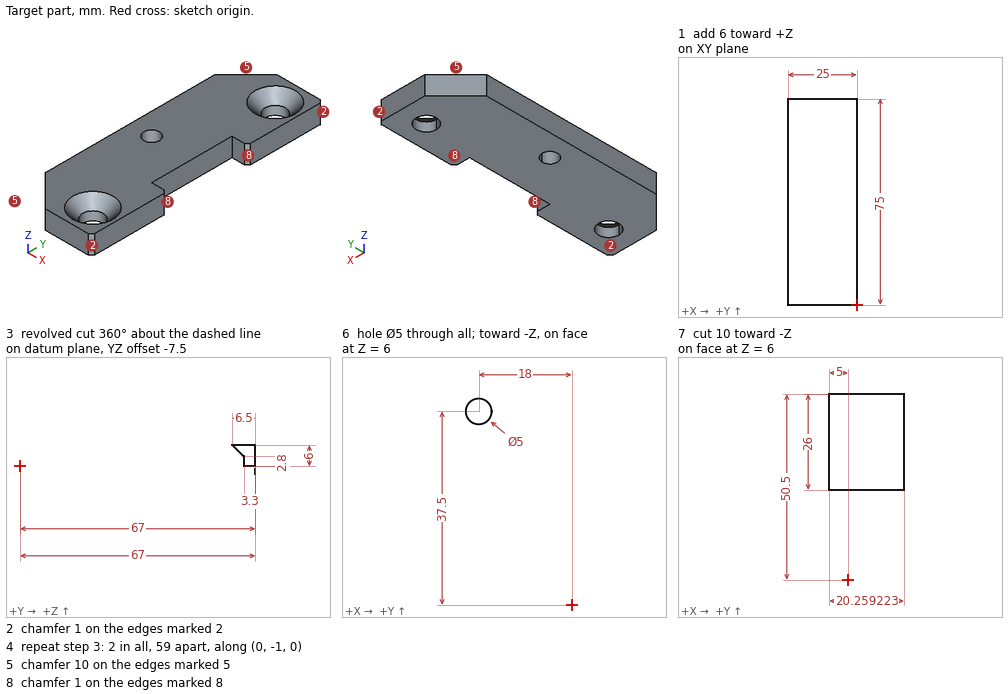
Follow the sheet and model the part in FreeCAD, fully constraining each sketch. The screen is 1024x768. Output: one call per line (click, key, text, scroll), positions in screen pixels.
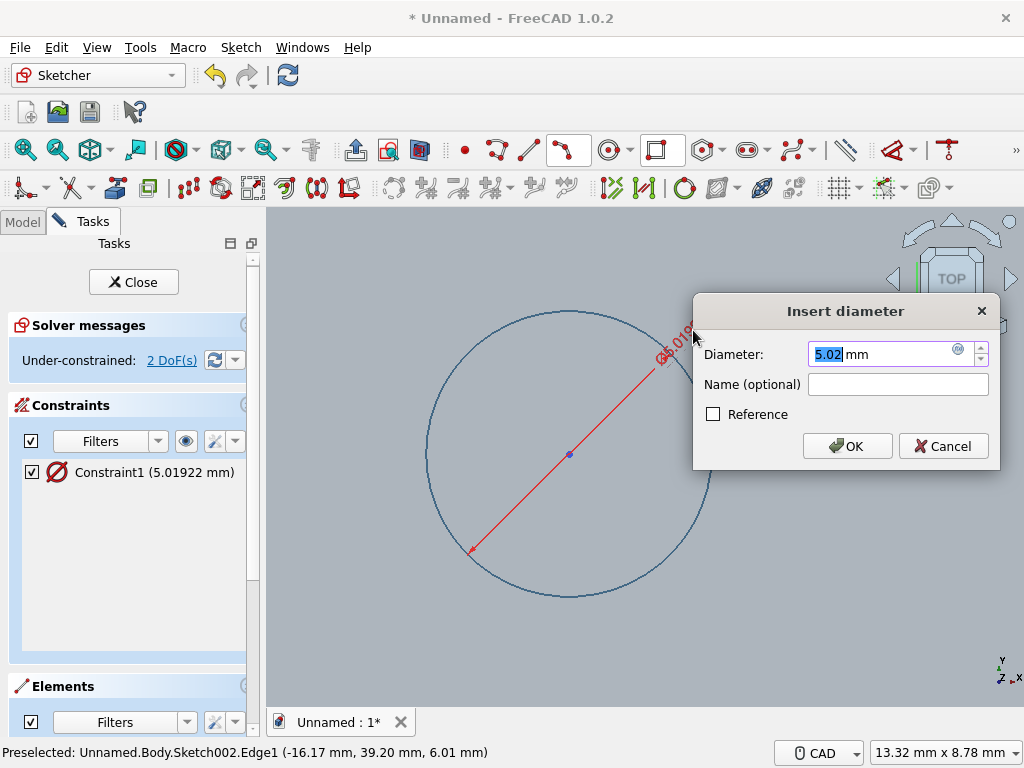
text(5)
key(Return)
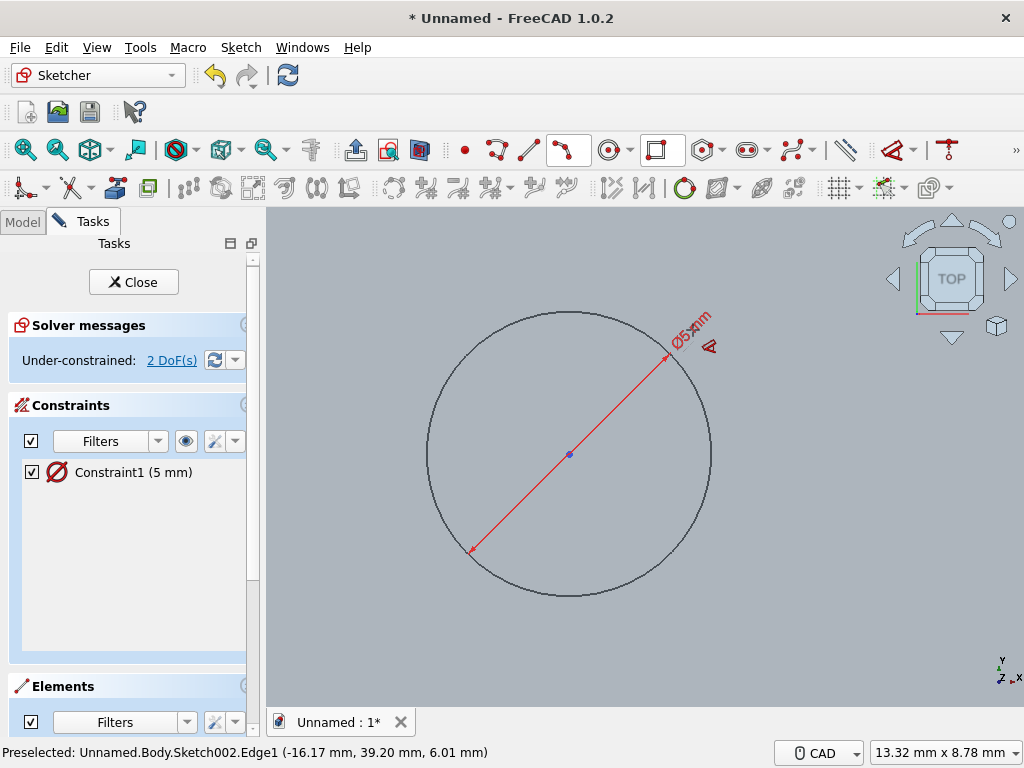
click(569, 454)
click(647, 420)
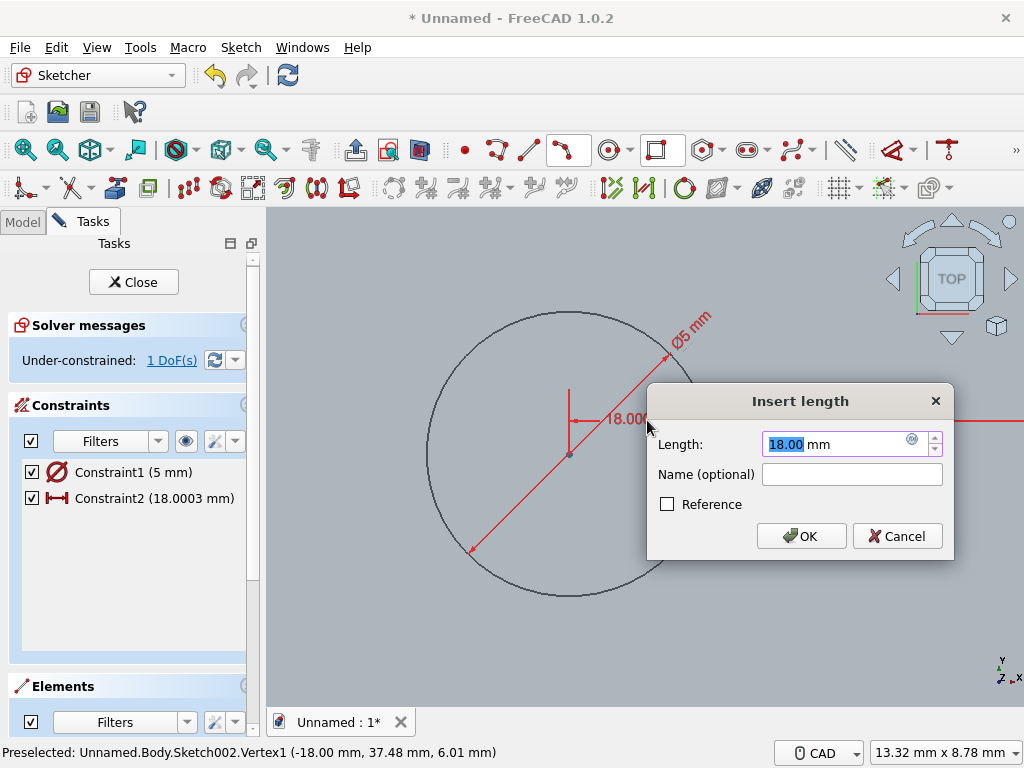
text(18)
key(Return)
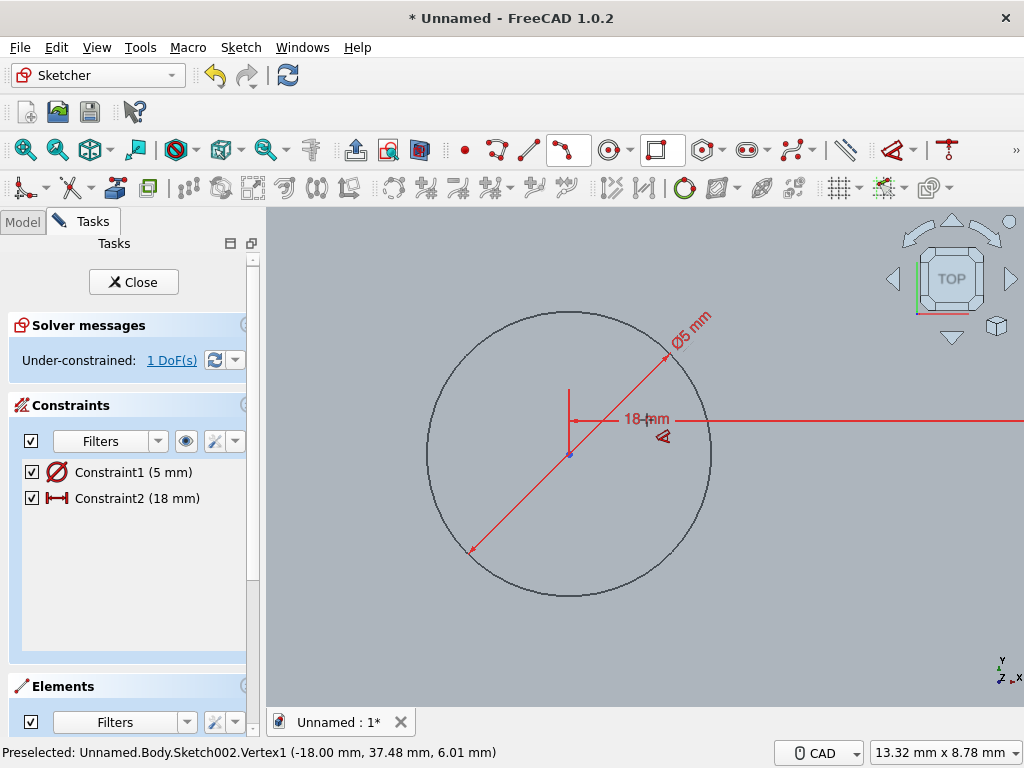
click(569, 454)
click(535, 567)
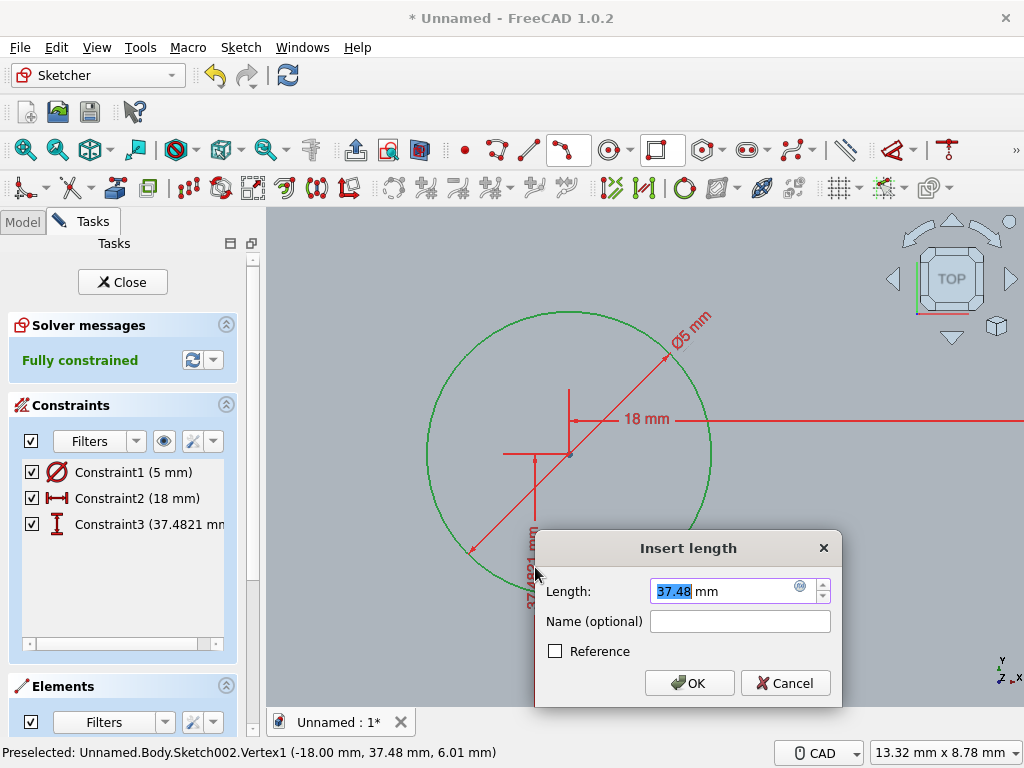
text(37.5)
key(Return)
key(Escape)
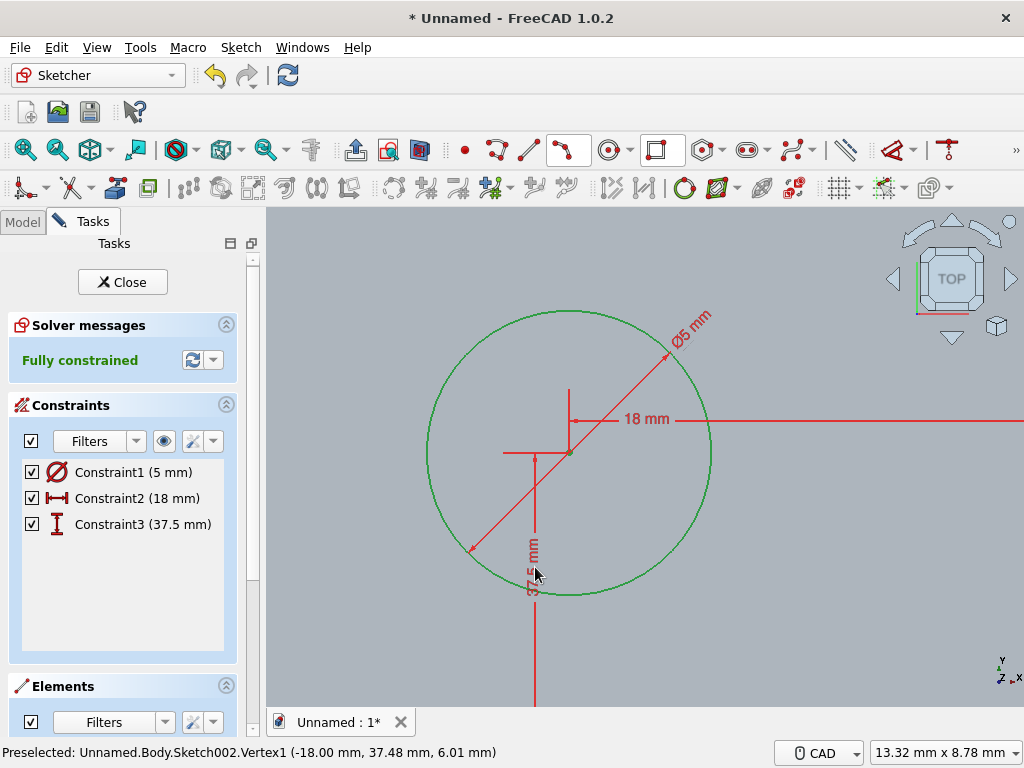
click(123, 282)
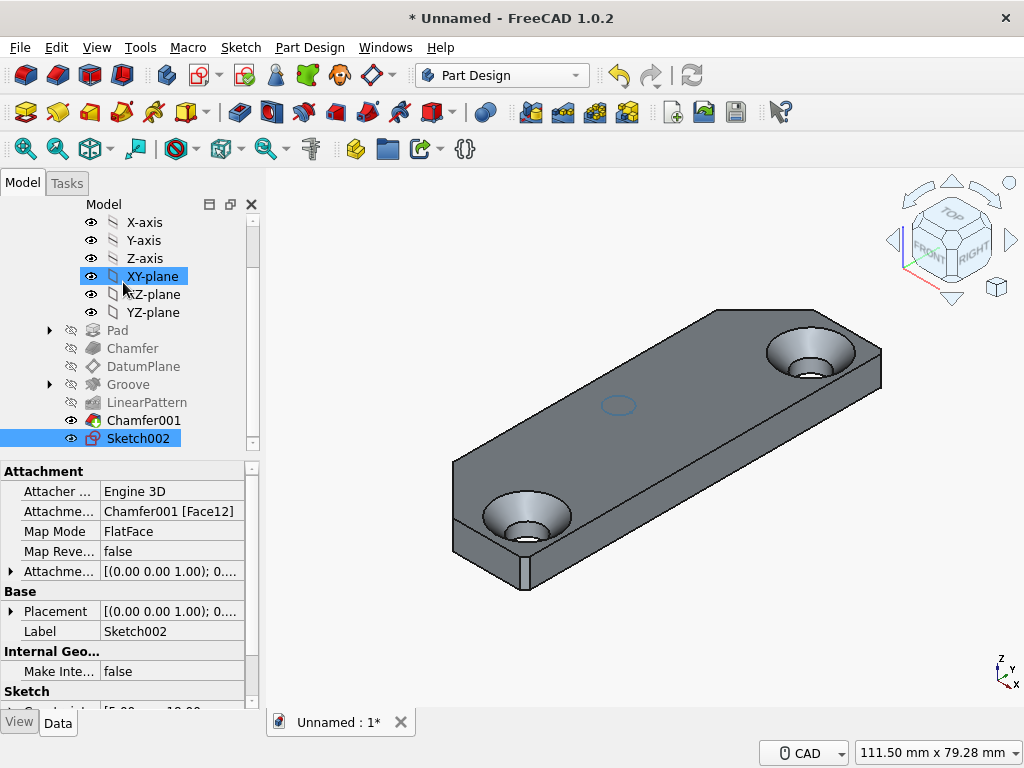
click(272, 112)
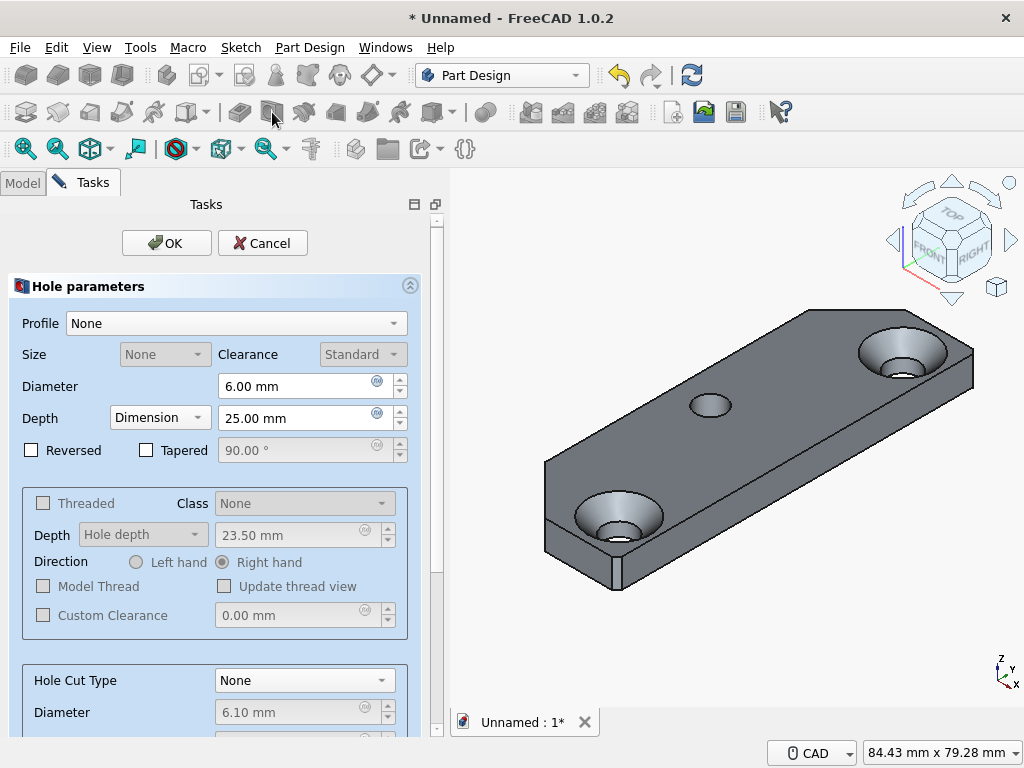
triple_click(305, 386)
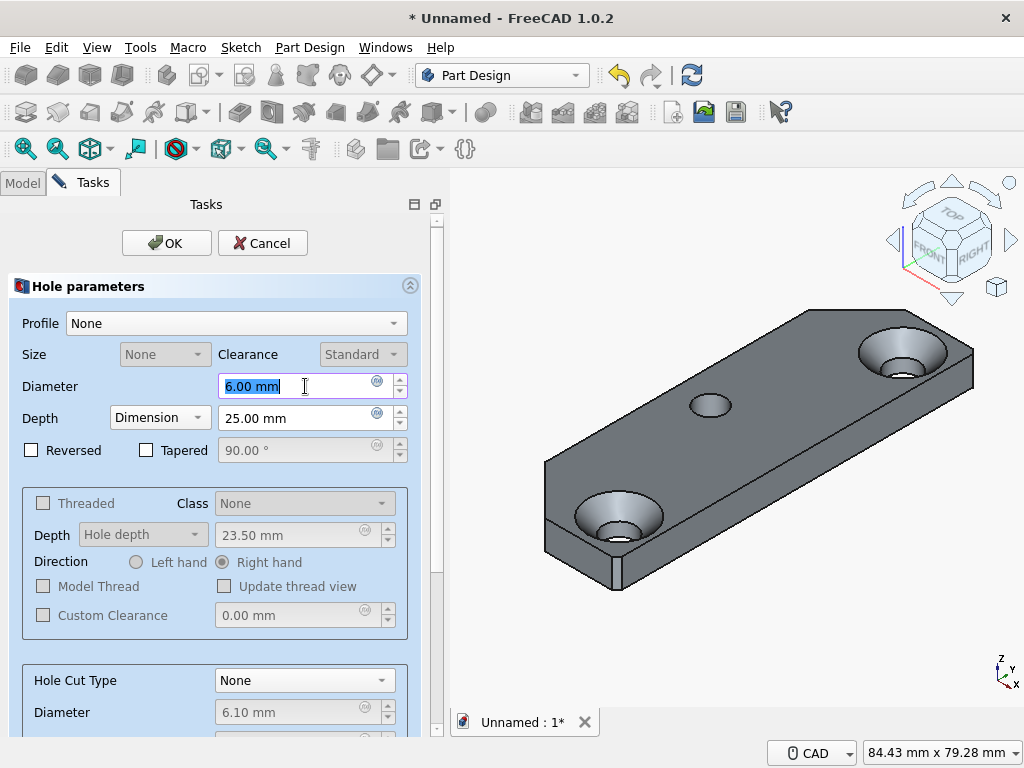
text(5)
key(Tab)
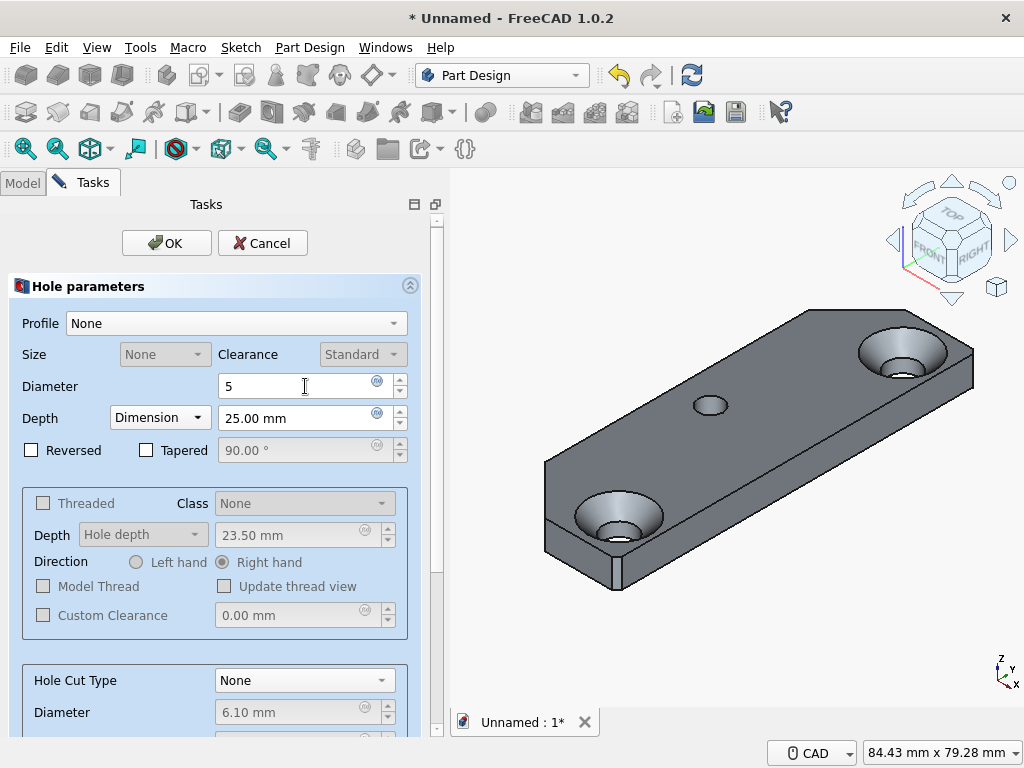
click(161, 418)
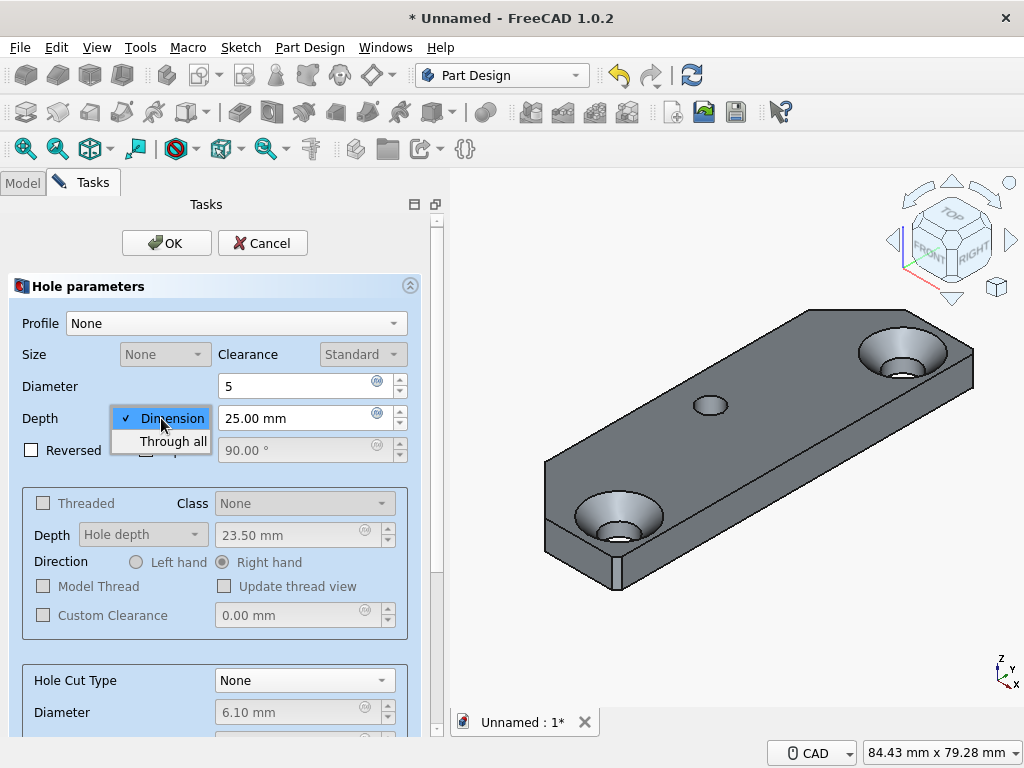
click(160, 442)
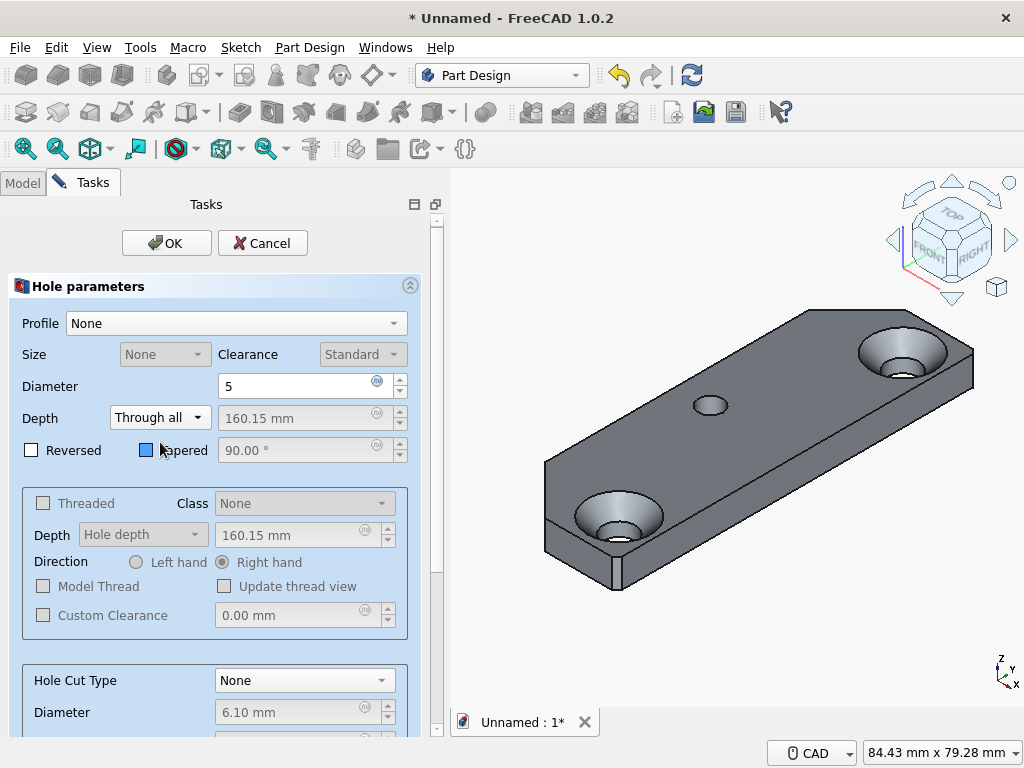
click(167, 243)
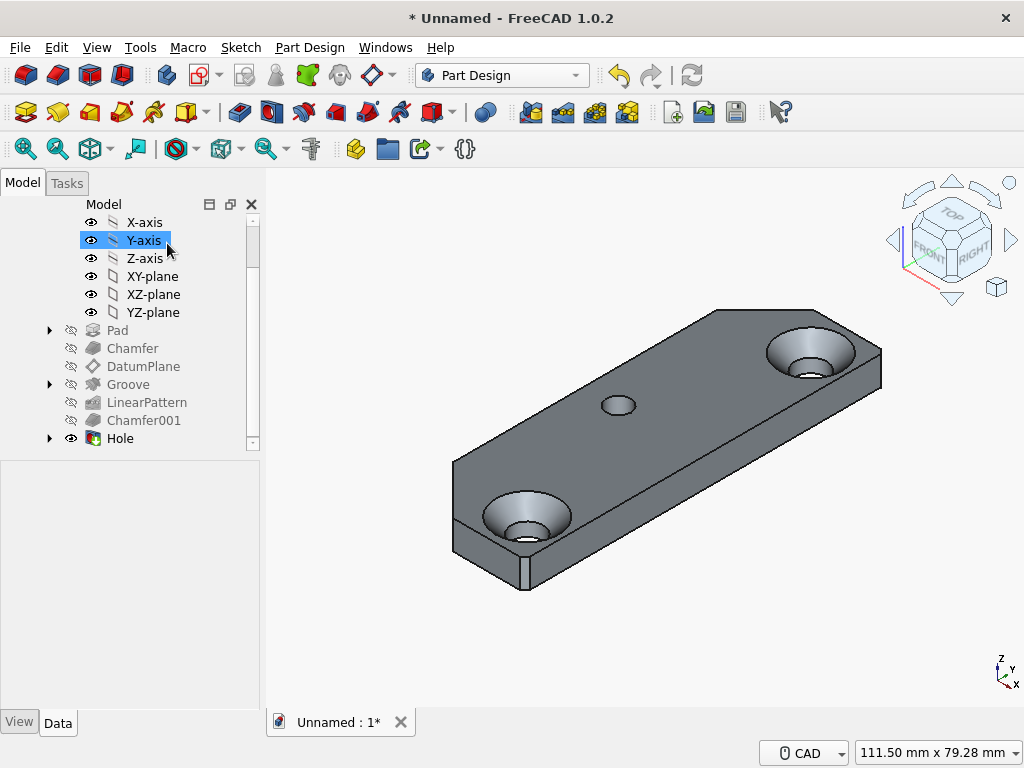
click(697, 390)